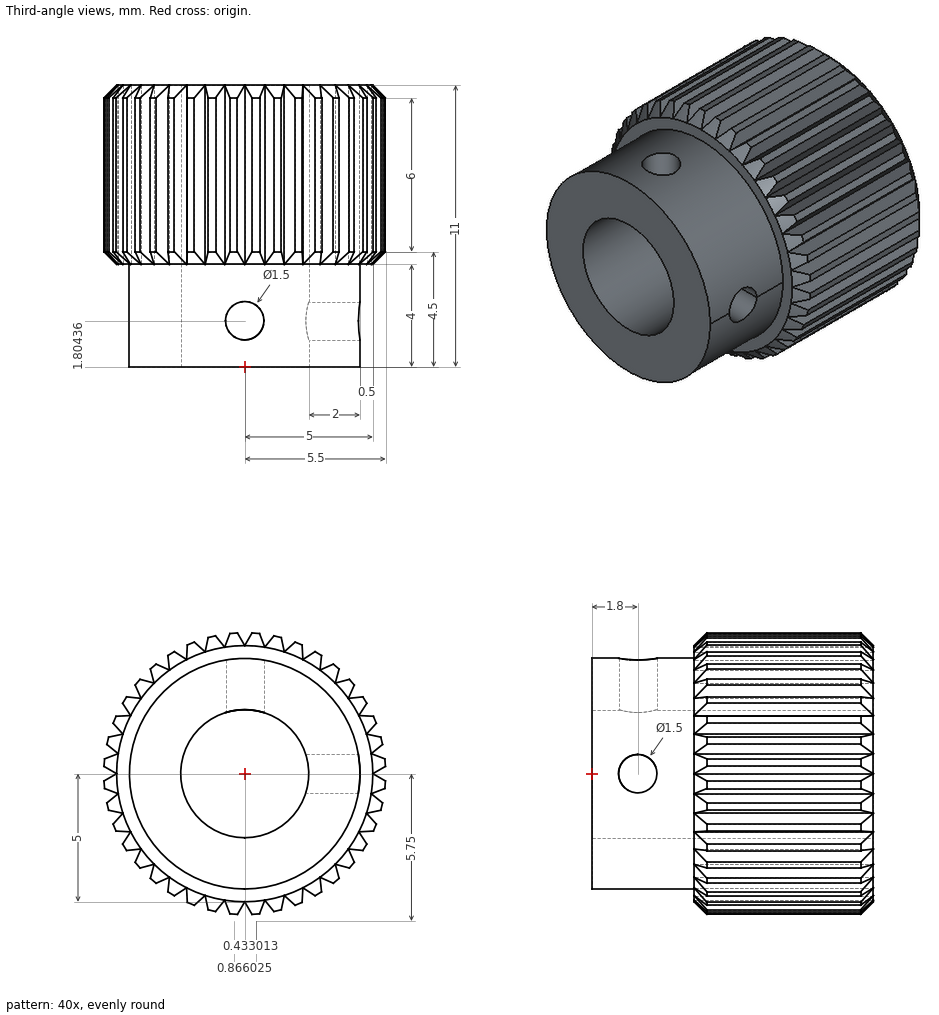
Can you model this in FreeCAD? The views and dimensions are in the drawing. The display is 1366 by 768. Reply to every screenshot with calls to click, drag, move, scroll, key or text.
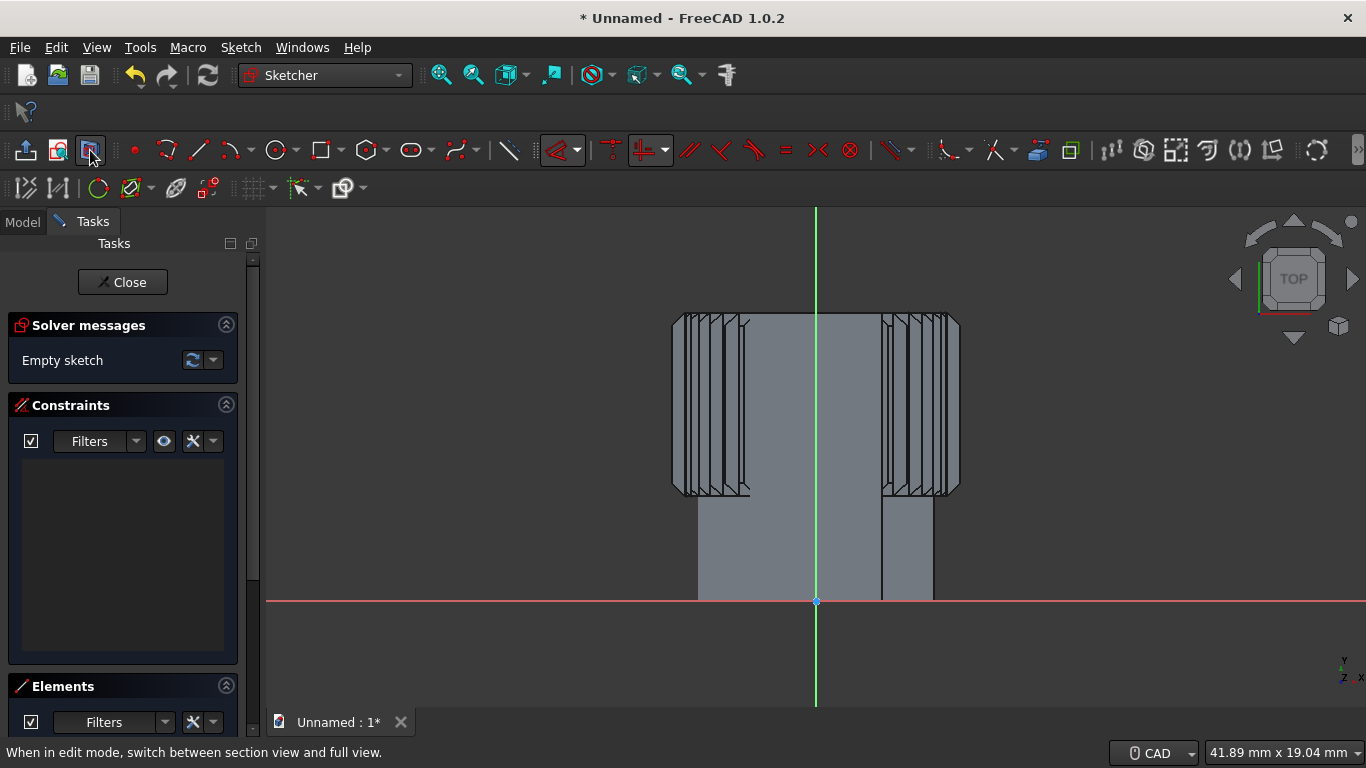
scroll(833, 596, up, 8)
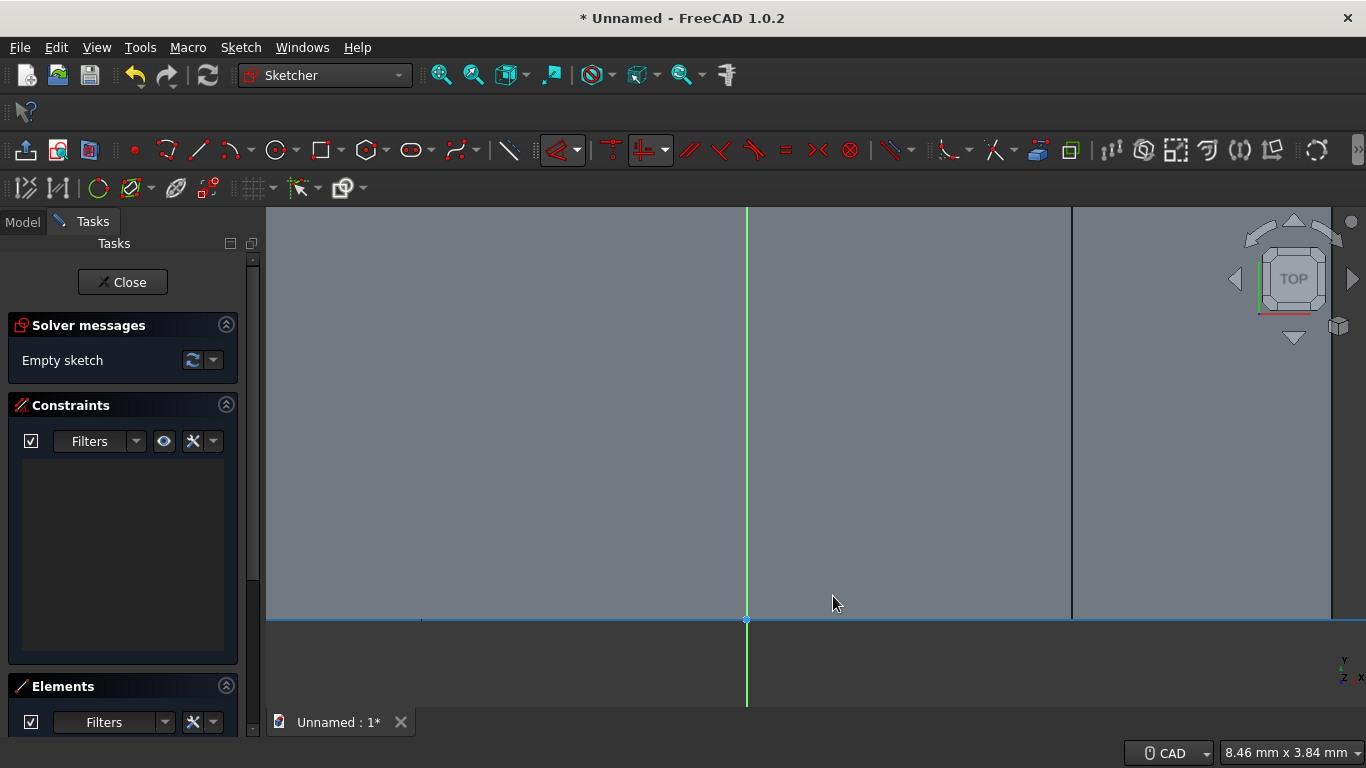
key(g)
key(c)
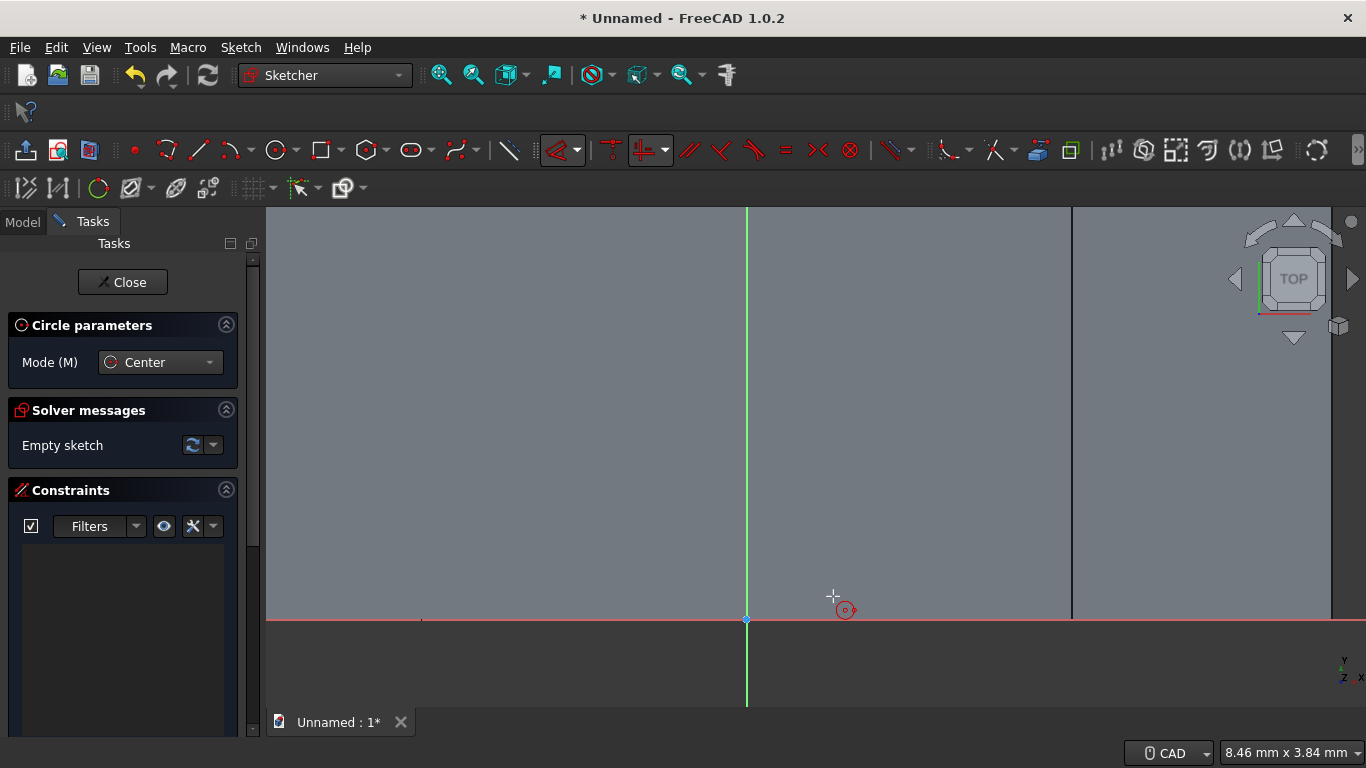
click(747, 385)
move(816, 316)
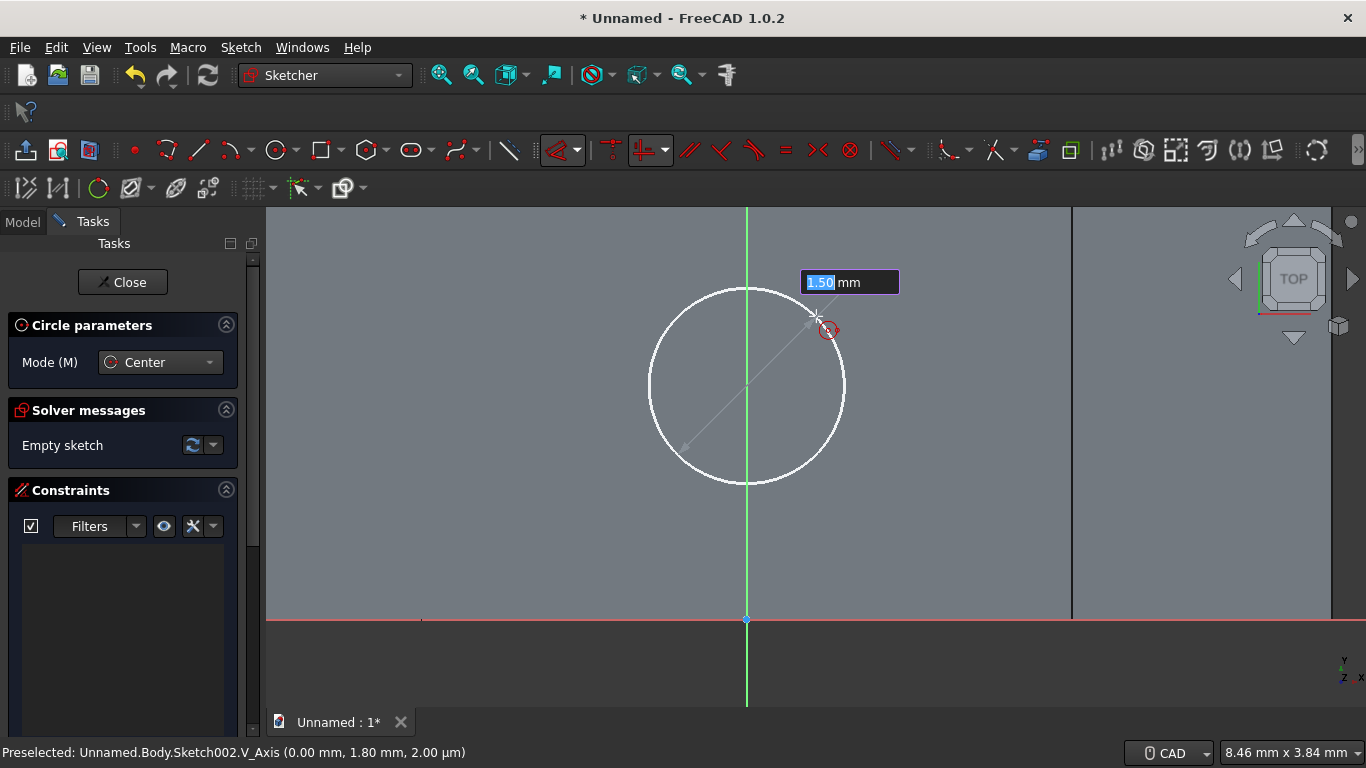
text(1.5)
key(Return)
key(Escape)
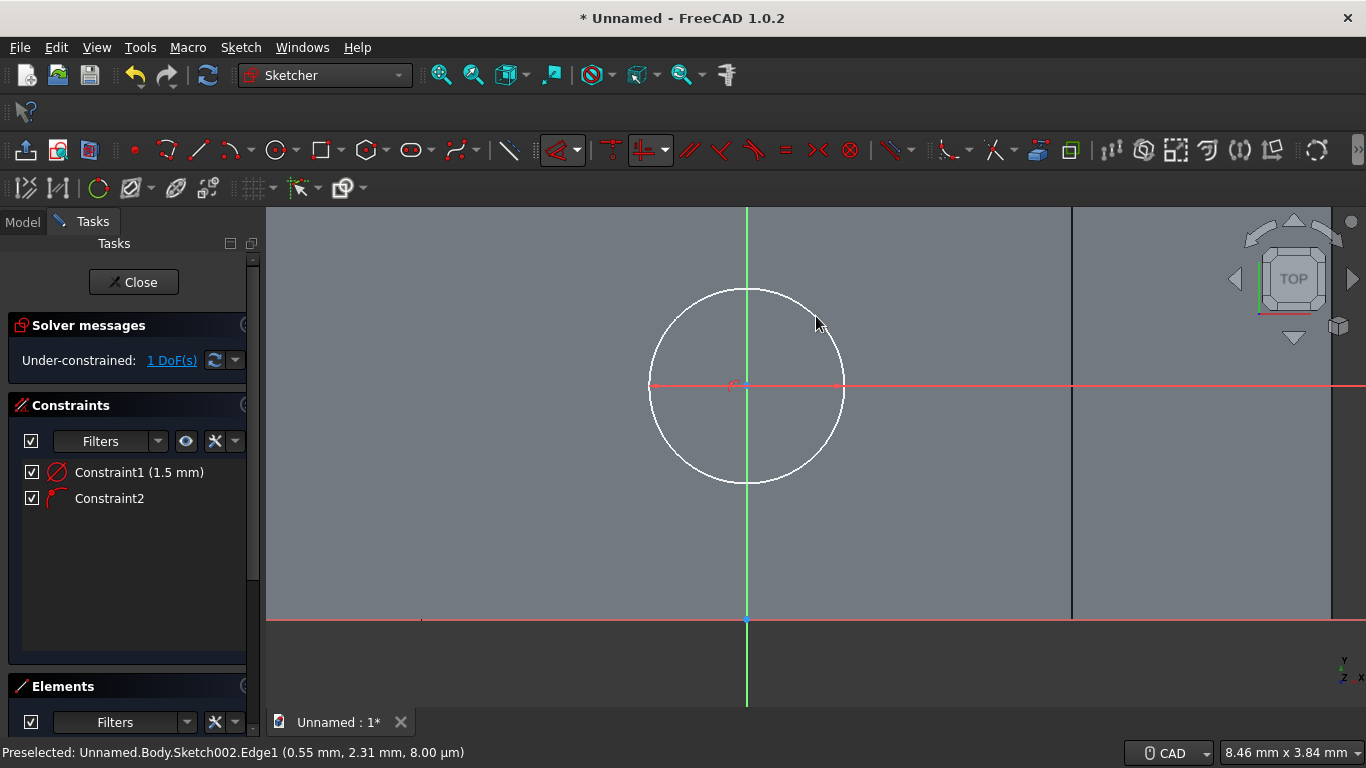
click(747, 386)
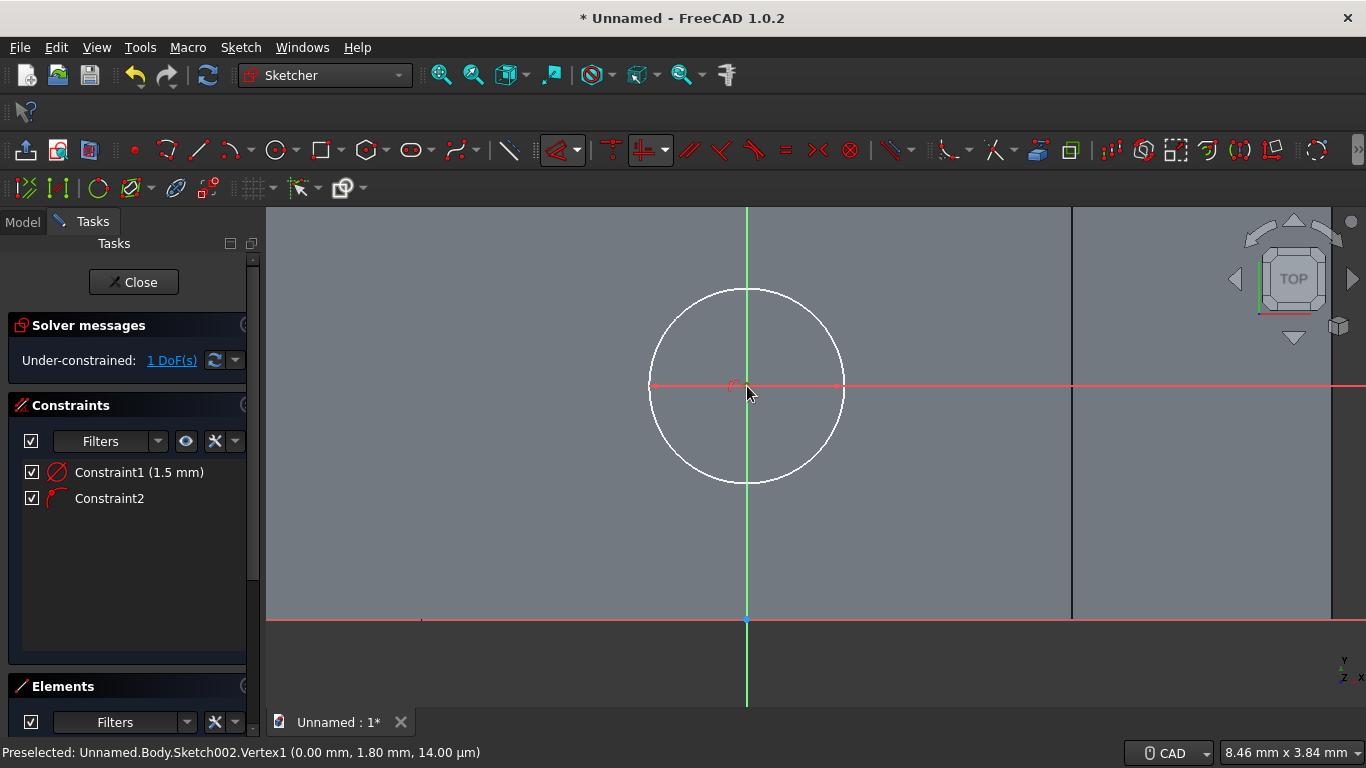
key(i)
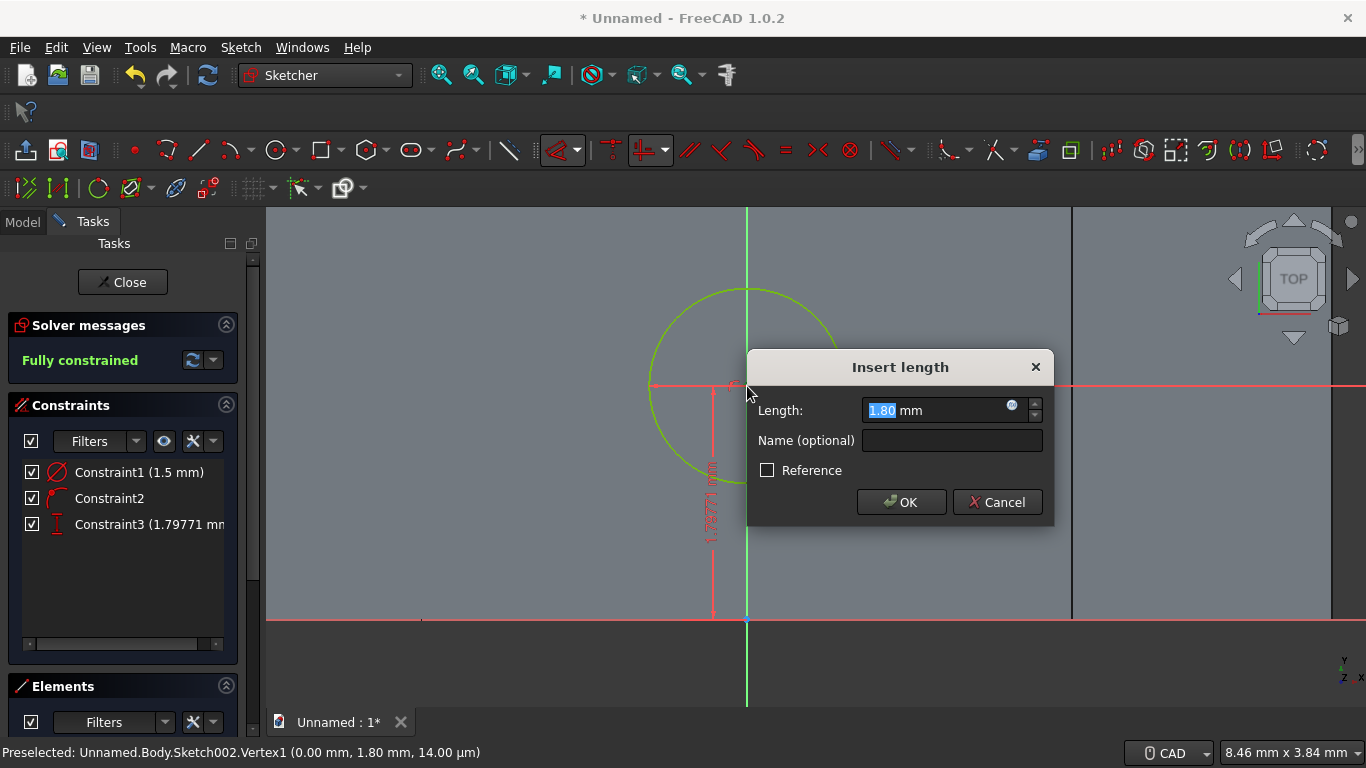
text(1.80436)
key(Return)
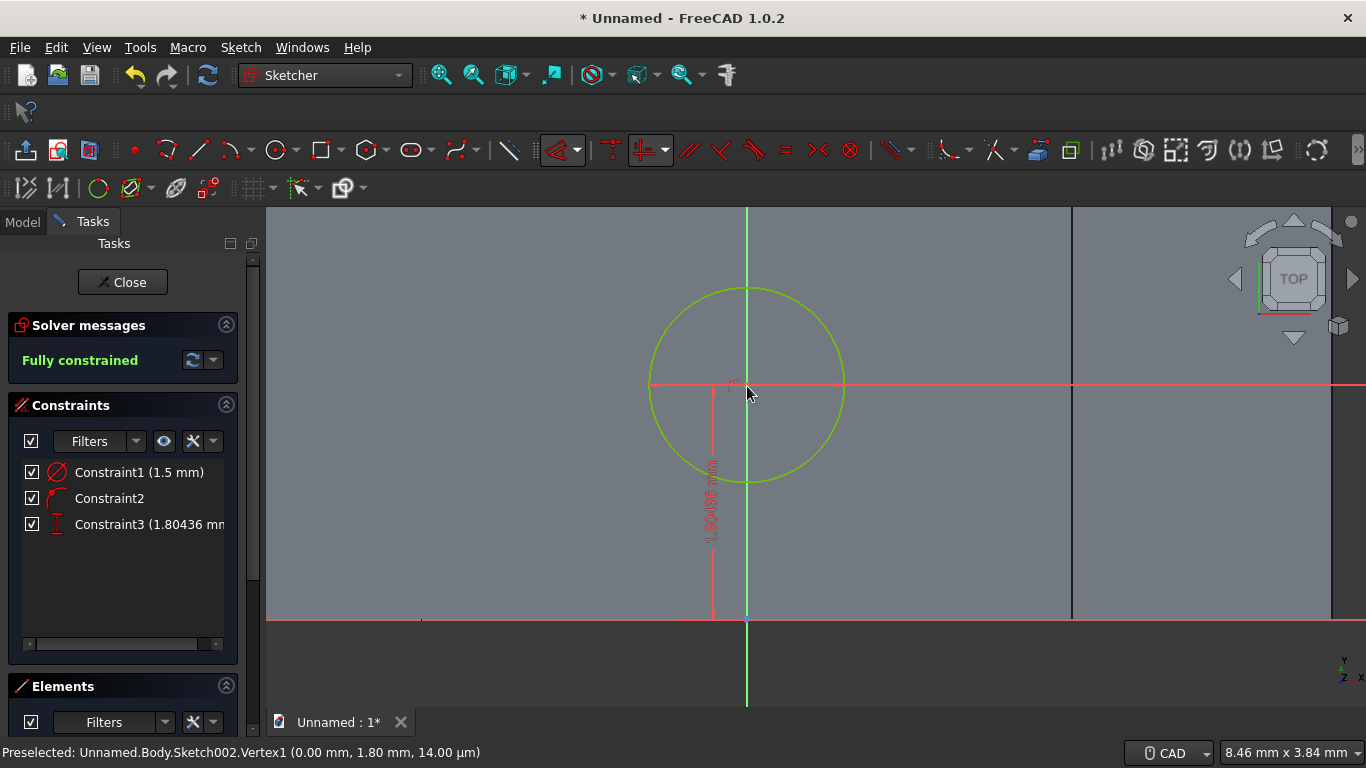
click(123, 282)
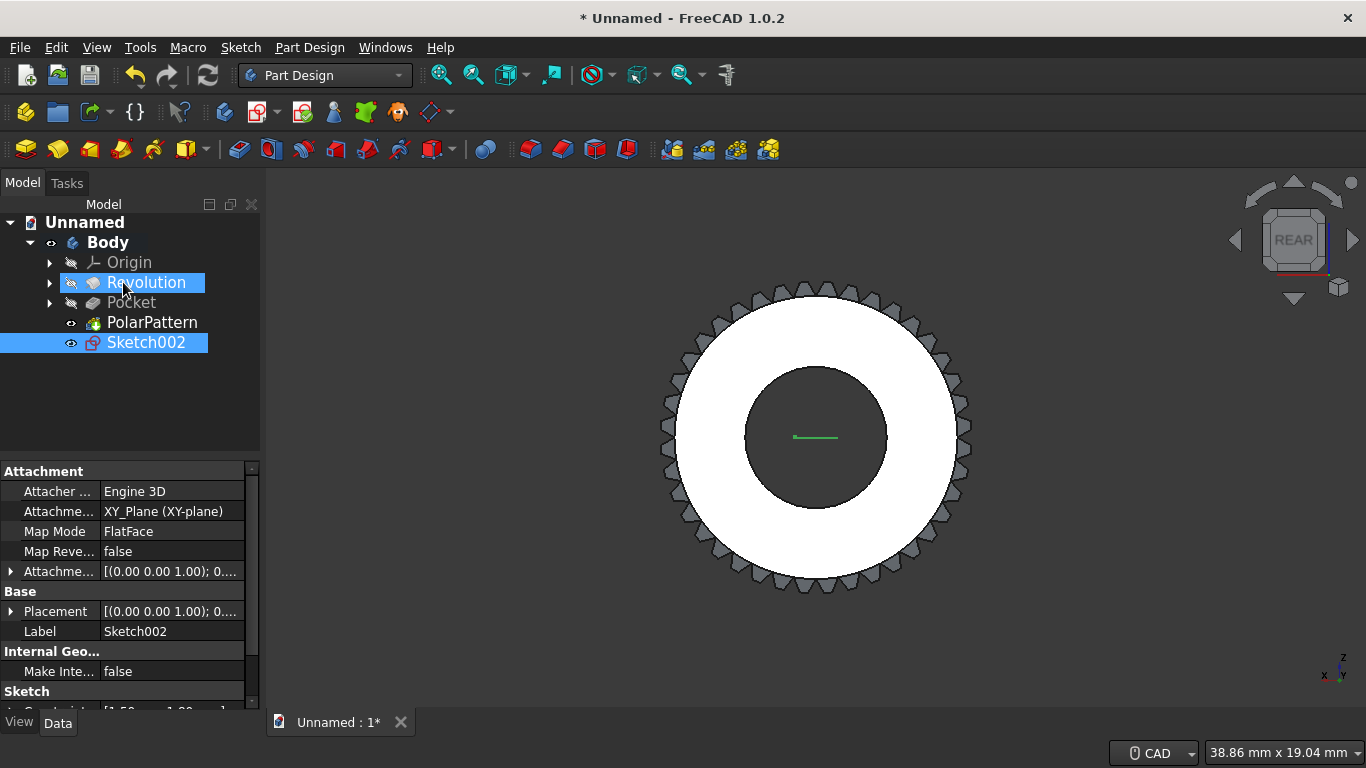
click(240, 150)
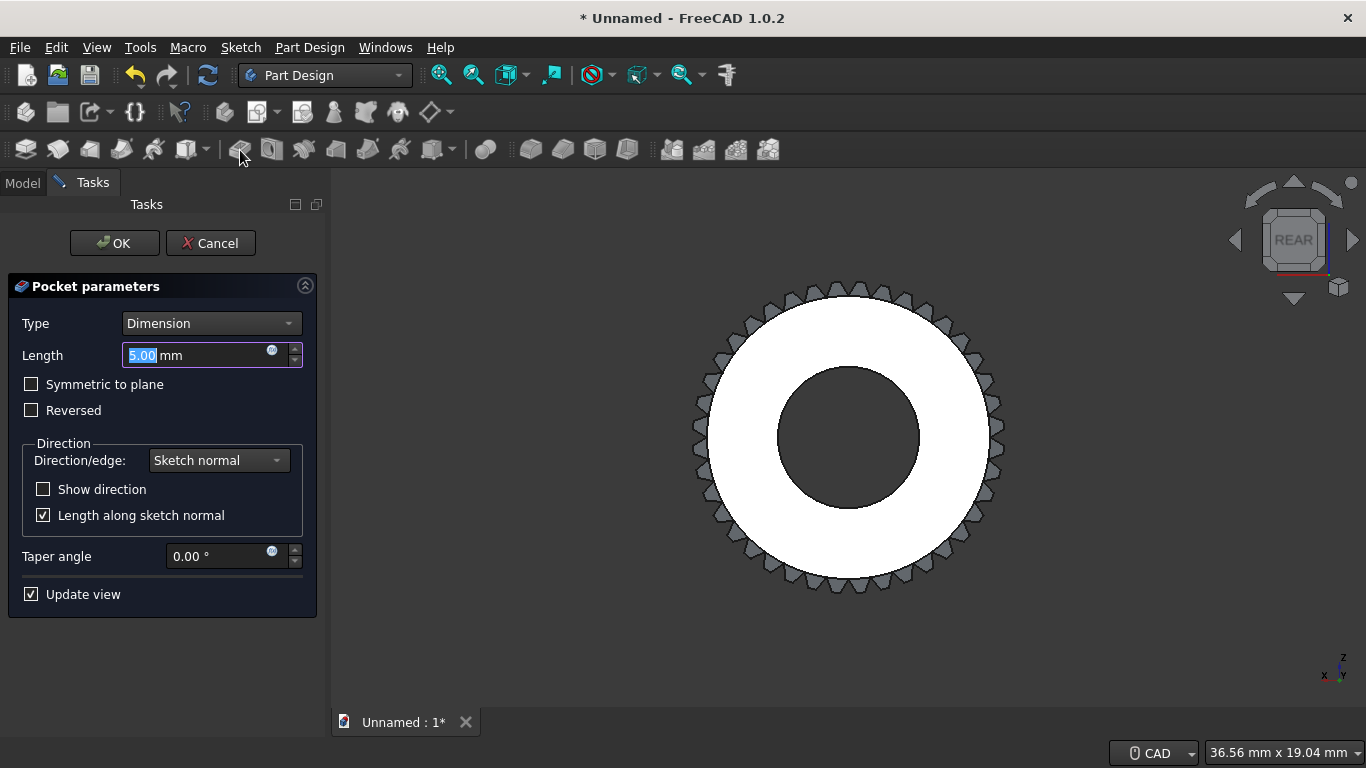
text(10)
key(Tab)